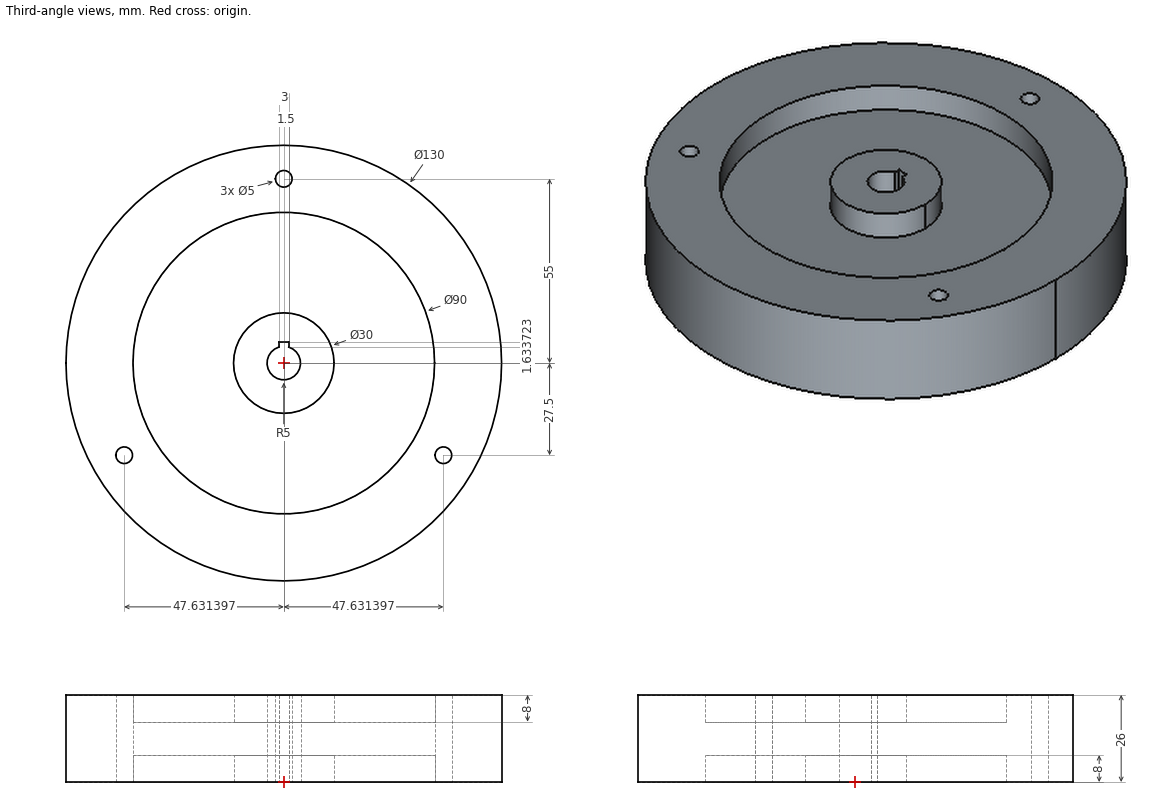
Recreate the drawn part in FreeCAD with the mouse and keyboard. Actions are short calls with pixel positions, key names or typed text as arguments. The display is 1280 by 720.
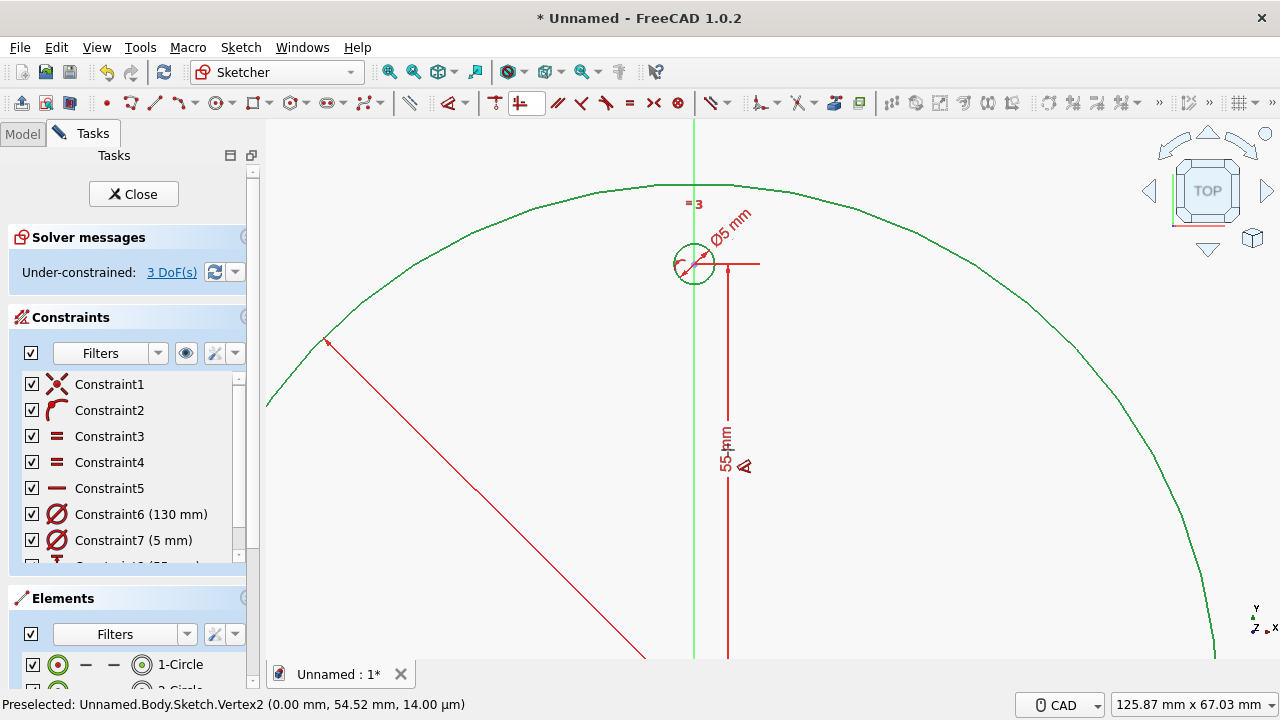
scroll(709, 252, down, 6)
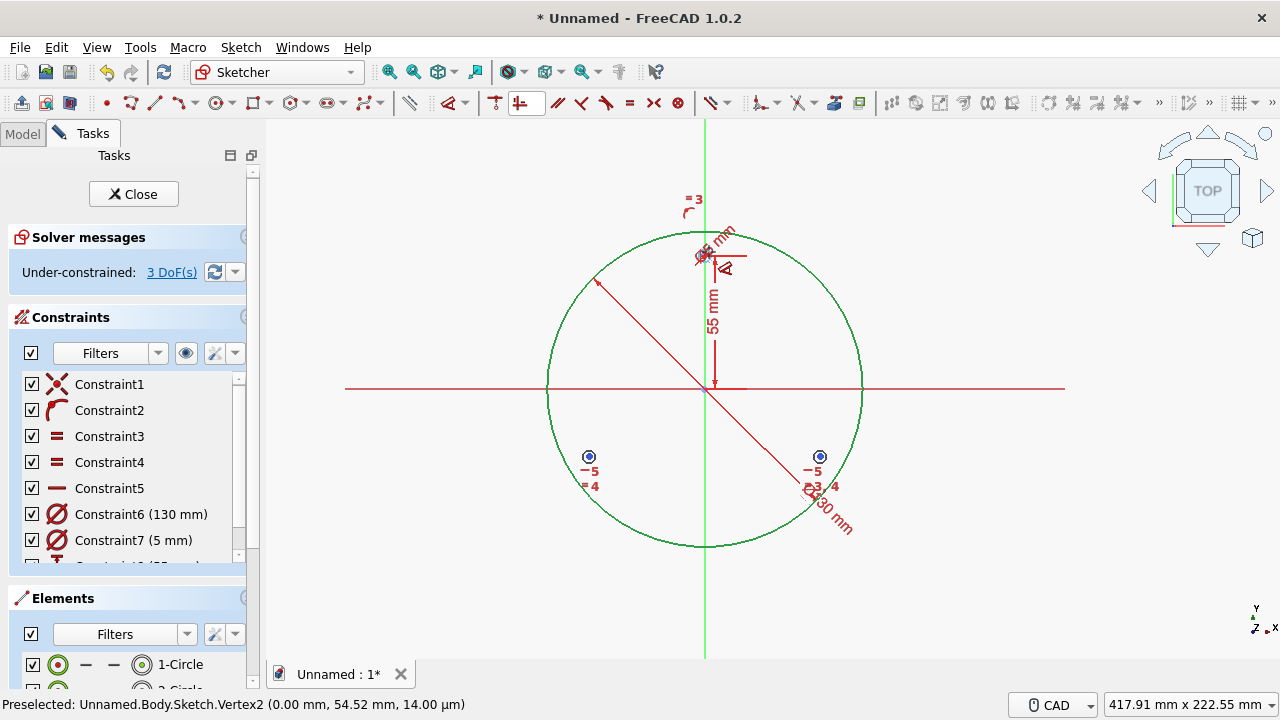
click(820, 457)
click(671, 423)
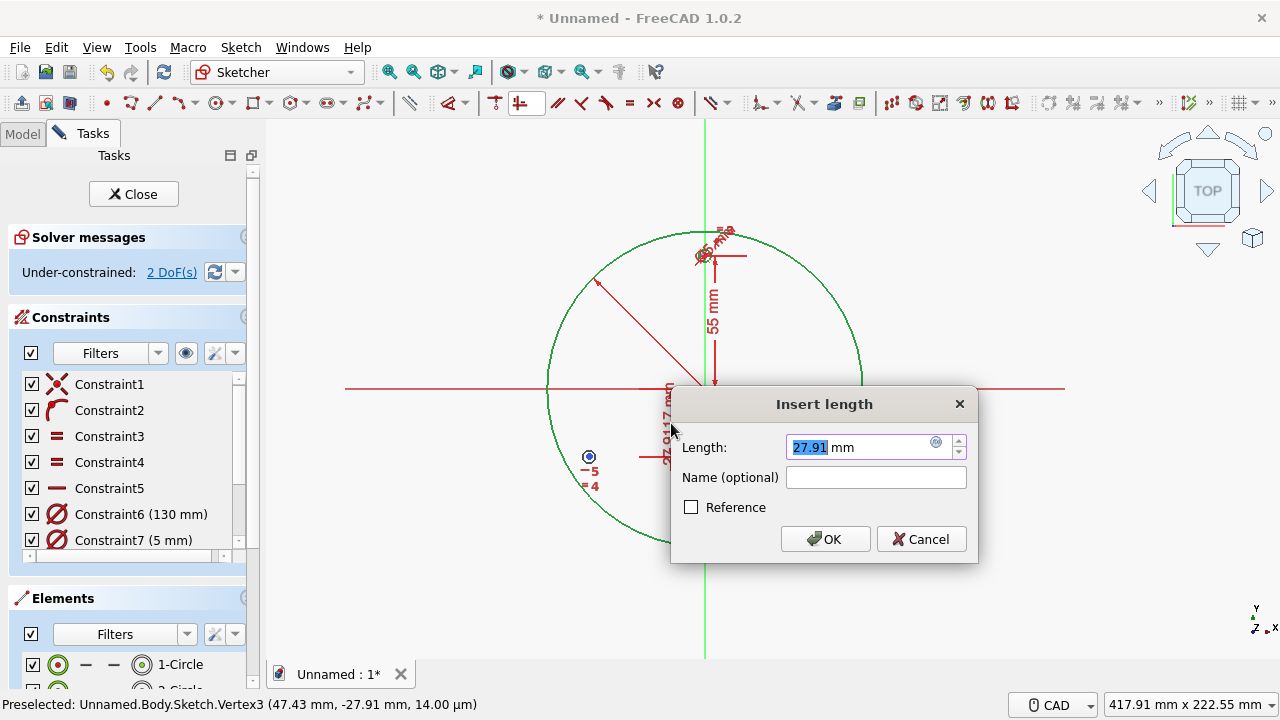
text(27.5)
key(Return)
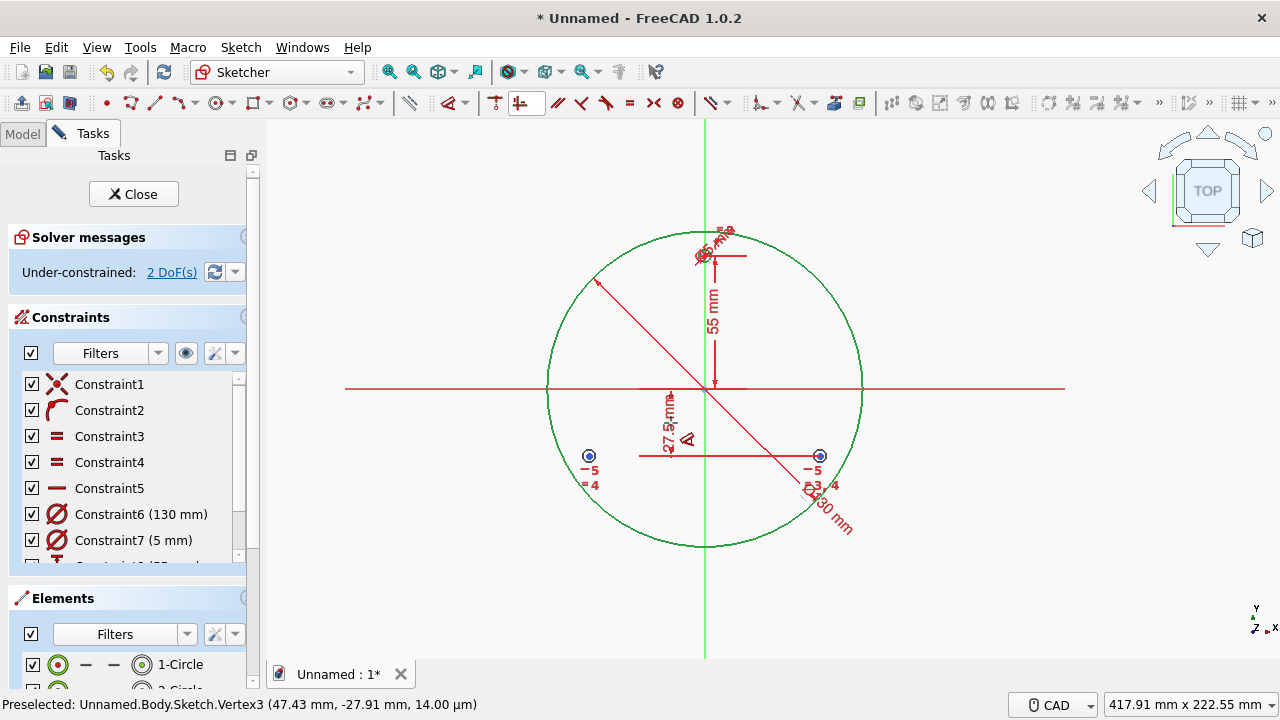
click(820, 456)
click(736, 490)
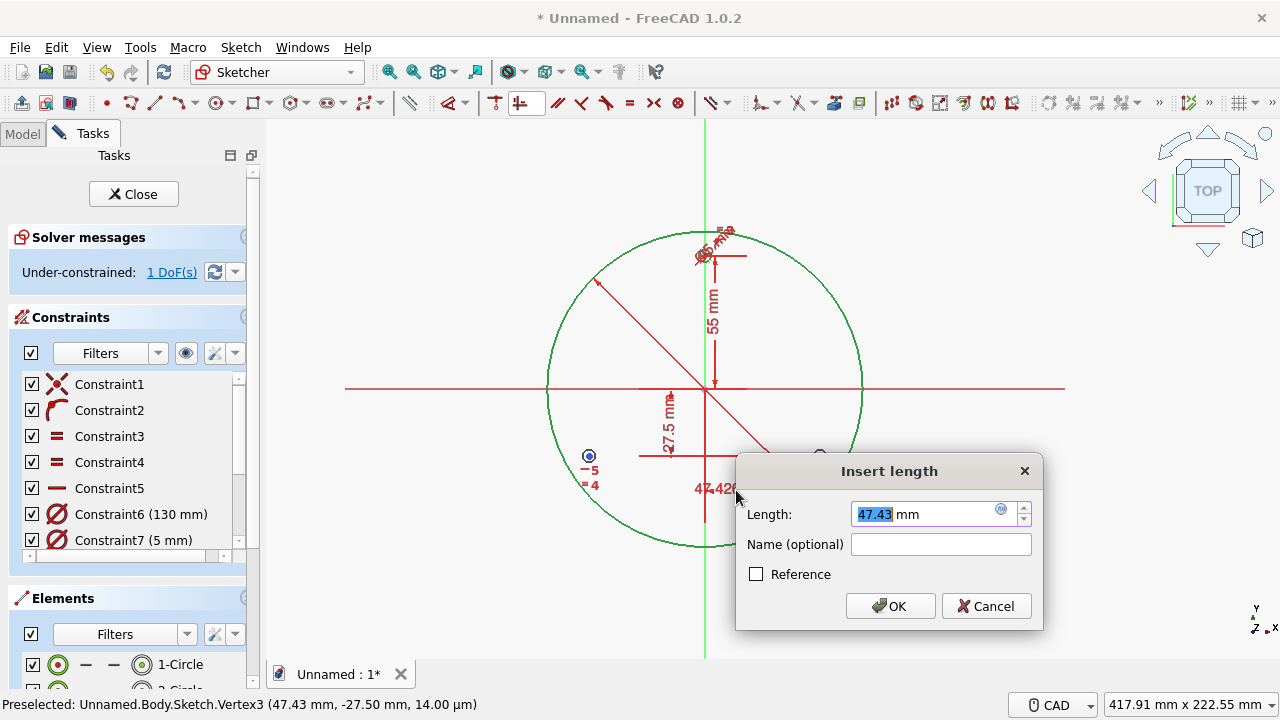
text(47.631397)
key(Return)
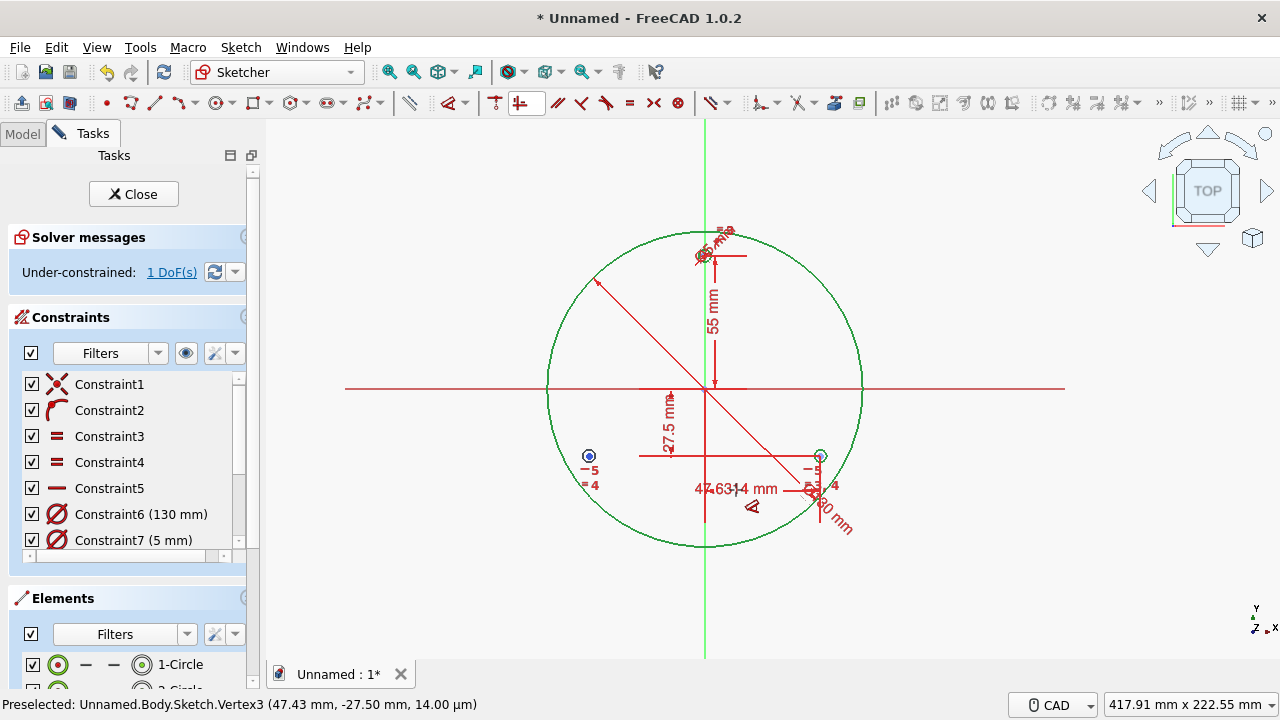
click(589, 456)
click(647, 490)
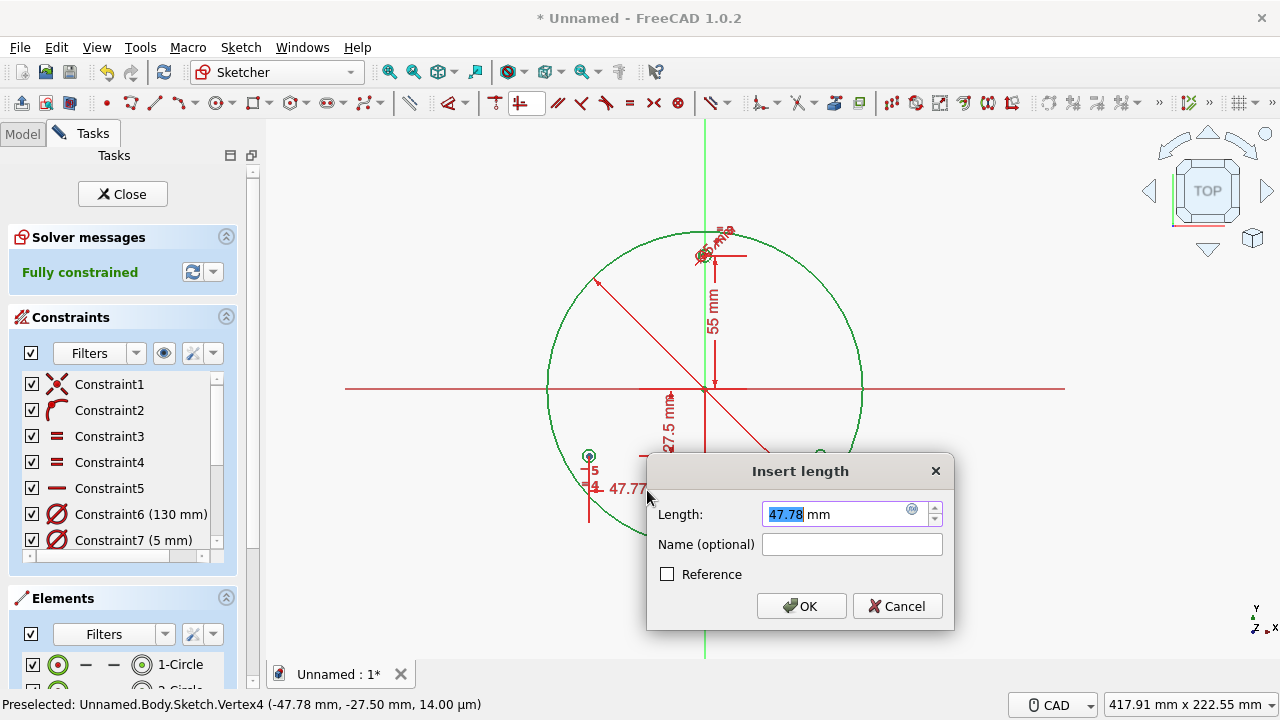
text(47.631397)
key(Return)
key(Escape)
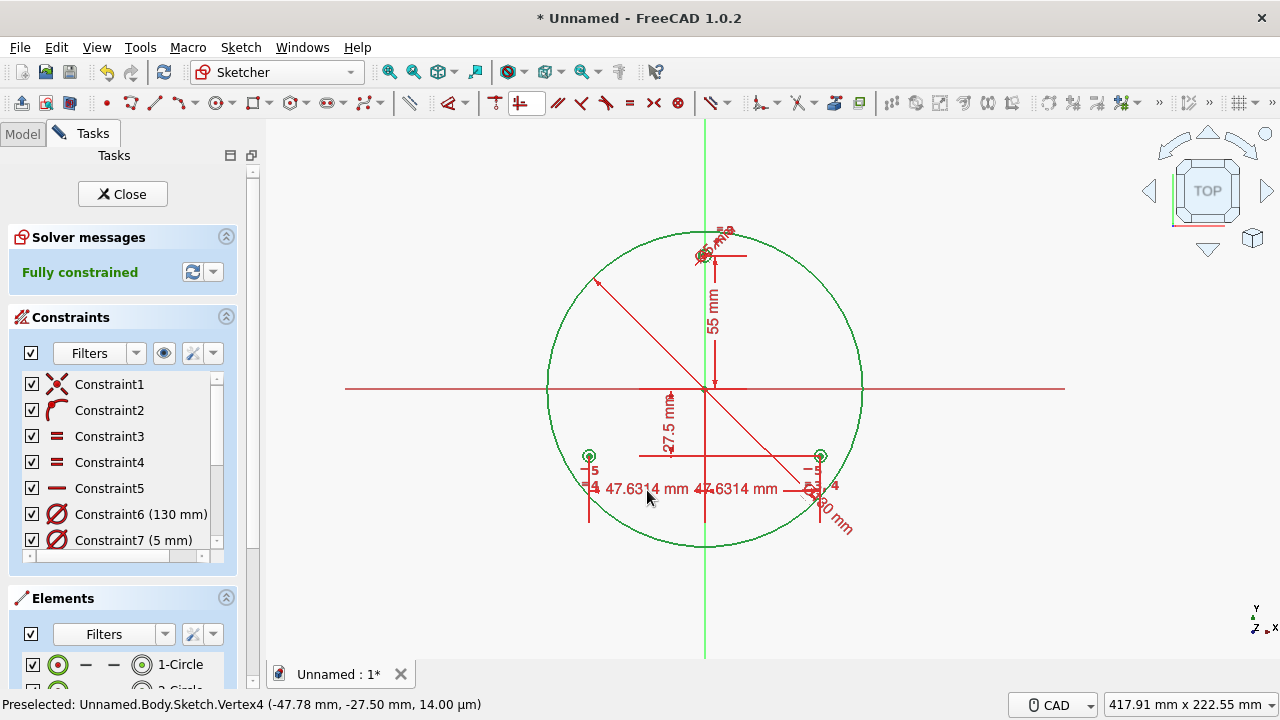
click(123, 194)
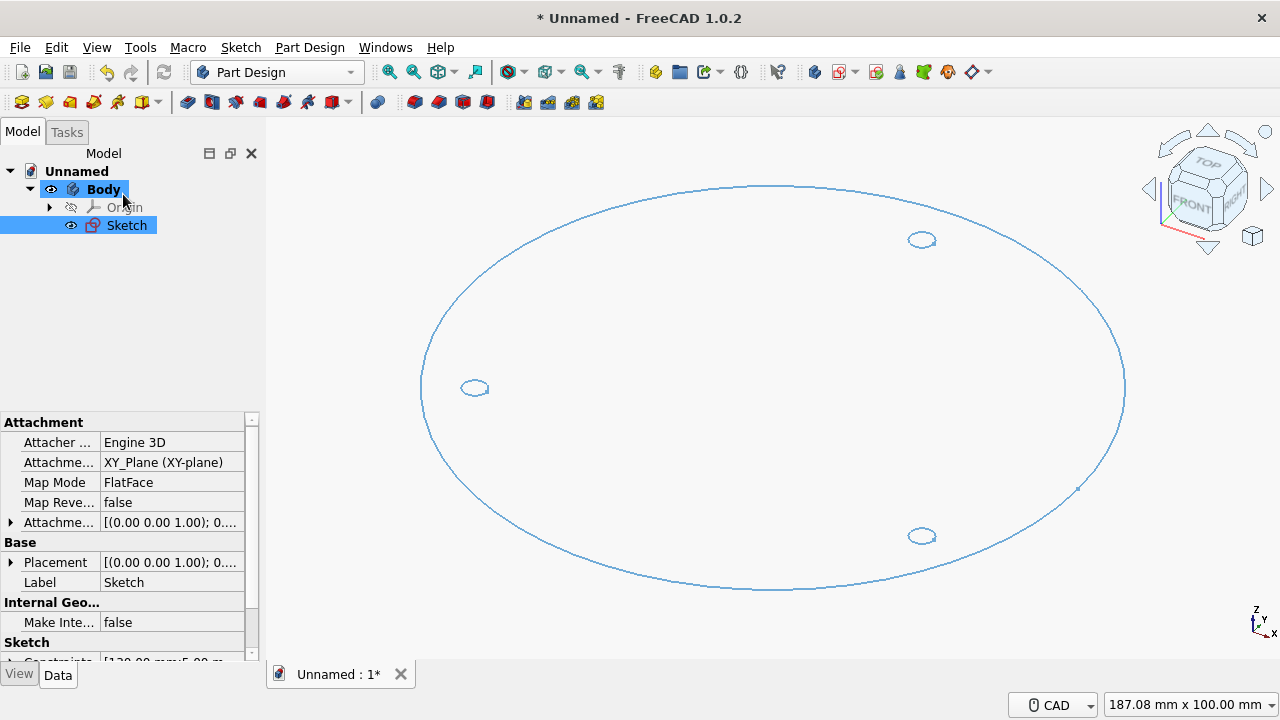
click(22, 102)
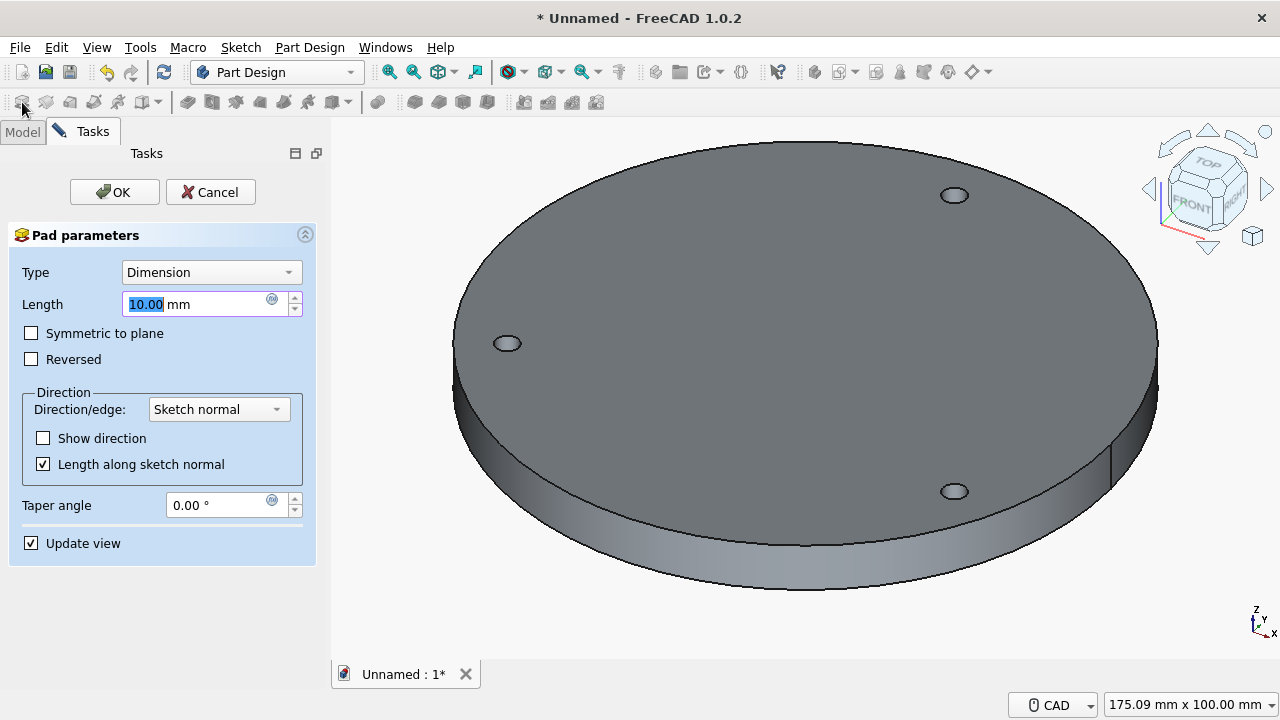
text(26)
key(Tab)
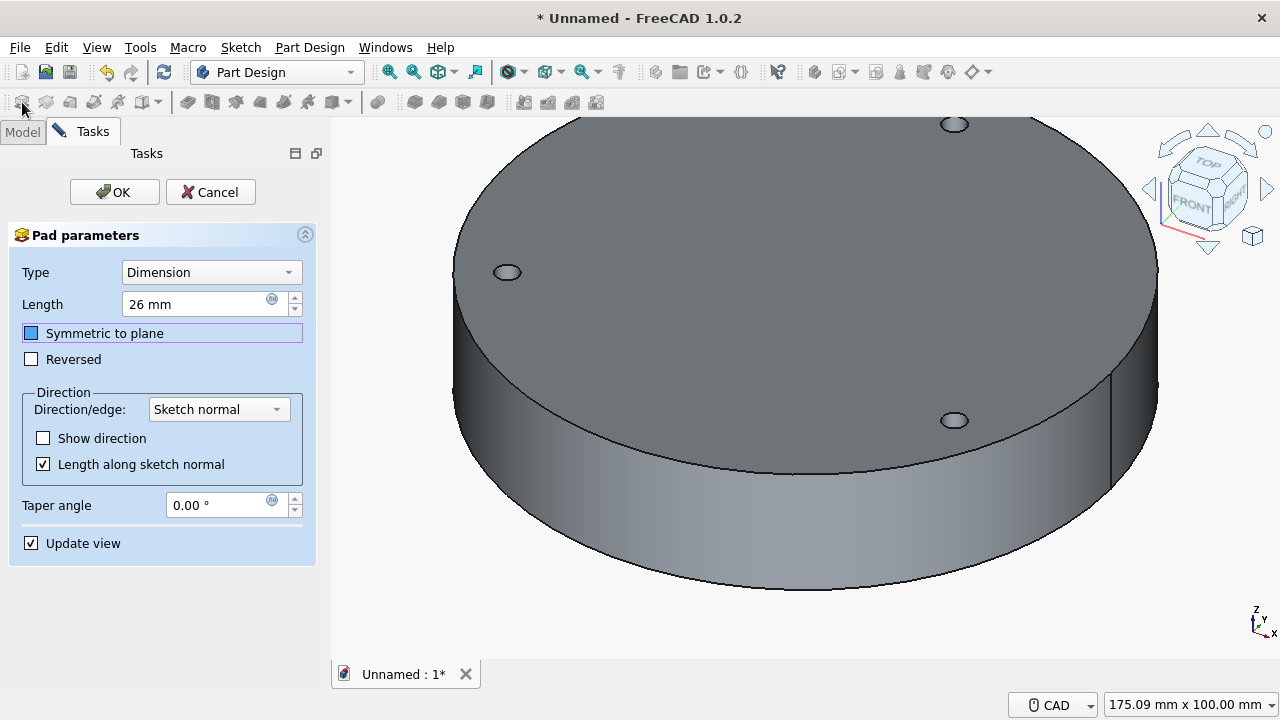
click(115, 192)